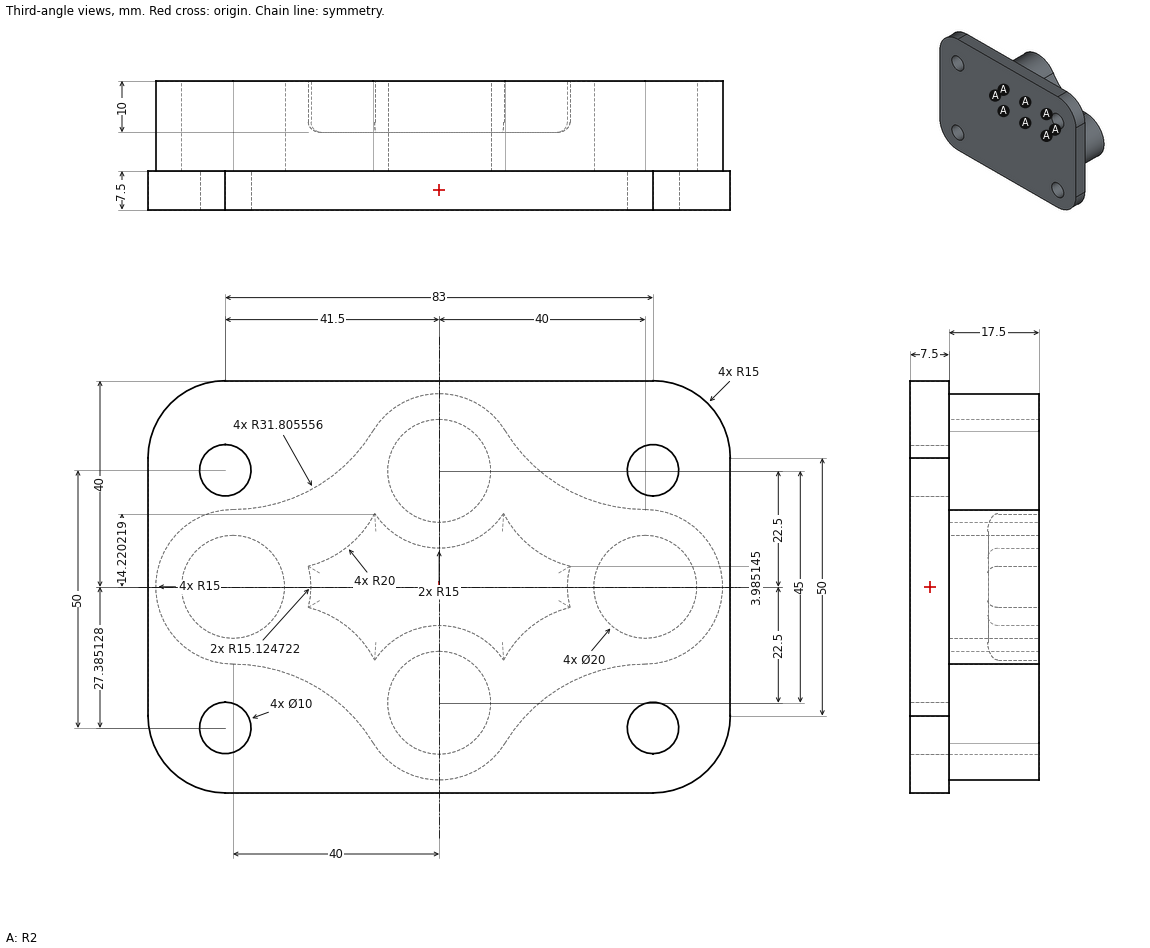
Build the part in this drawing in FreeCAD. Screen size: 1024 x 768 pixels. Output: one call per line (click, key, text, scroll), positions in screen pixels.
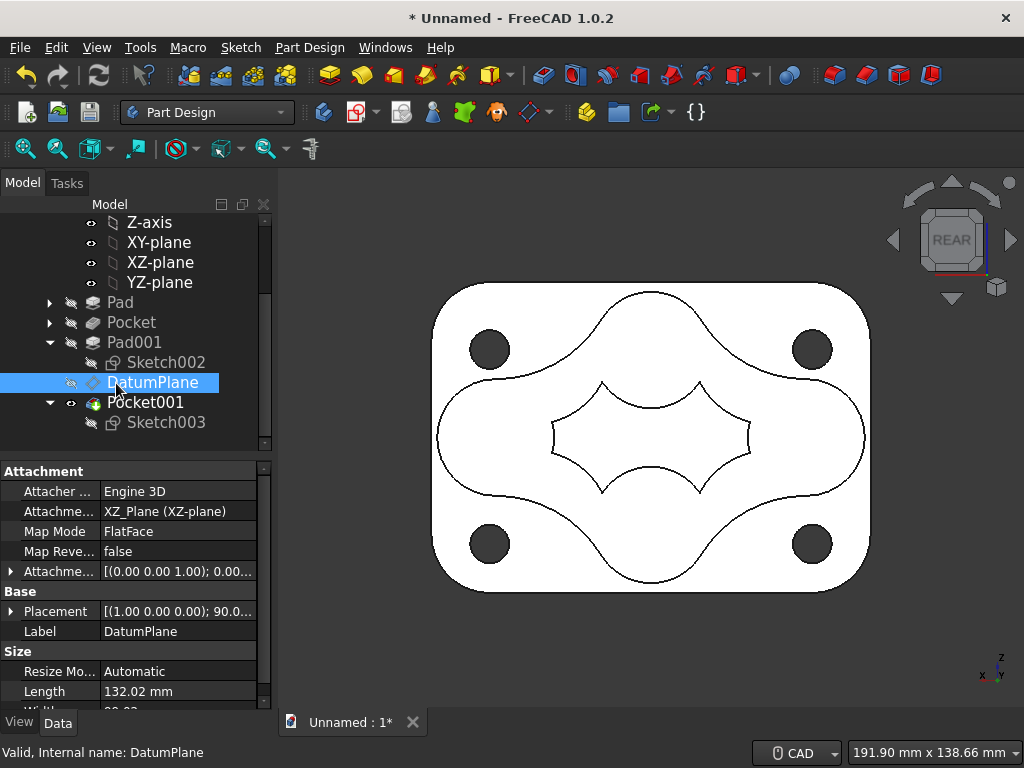
click(651, 353)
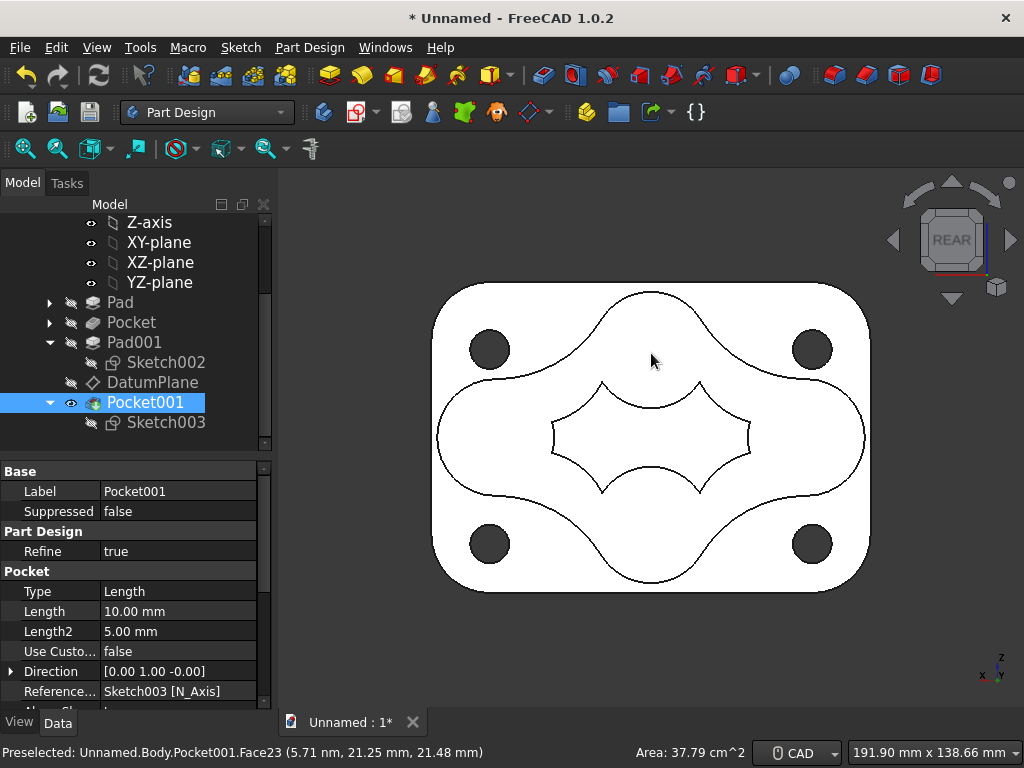
click(356, 112)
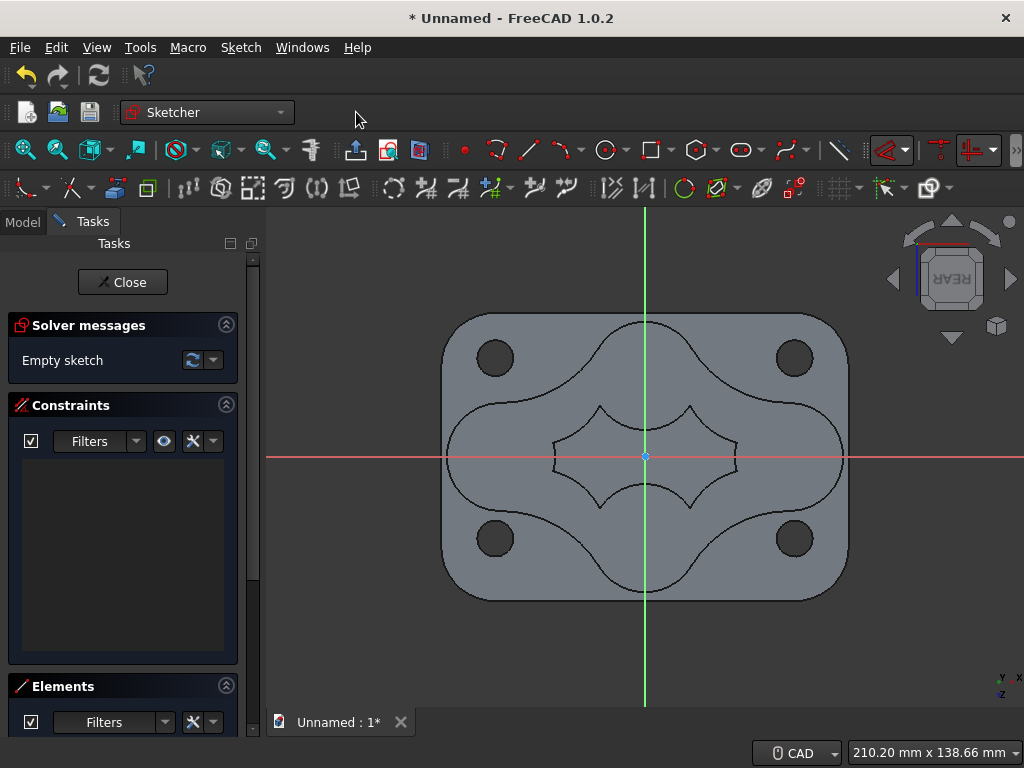
click(606, 150)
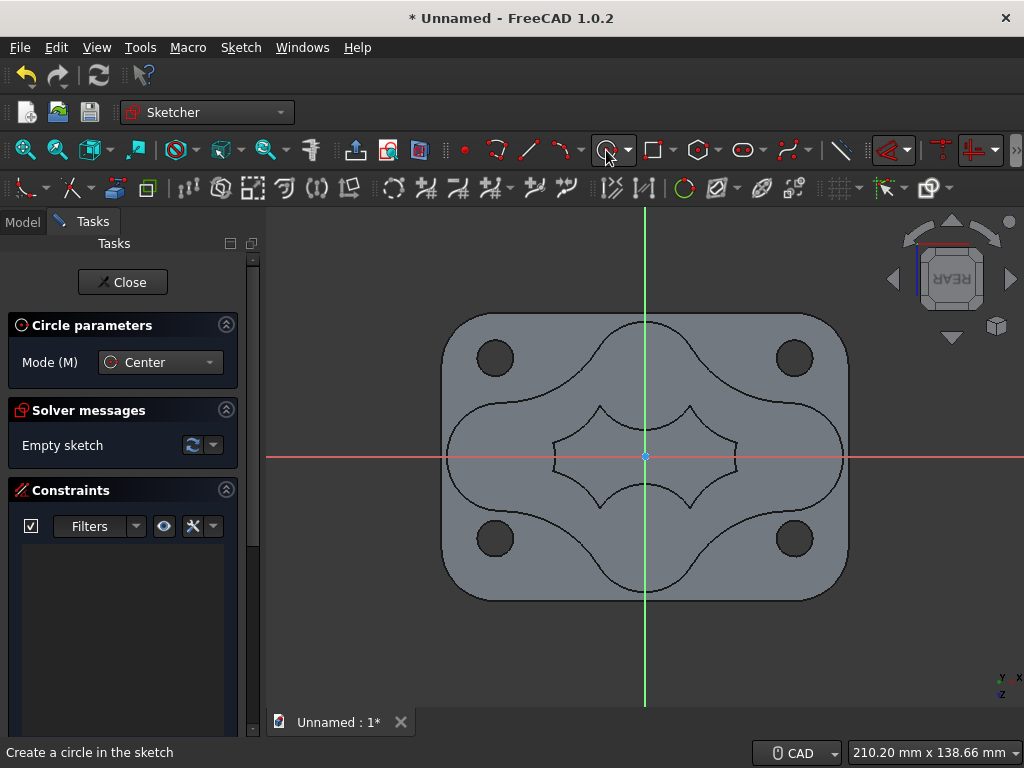
click(789, 457)
move(815, 432)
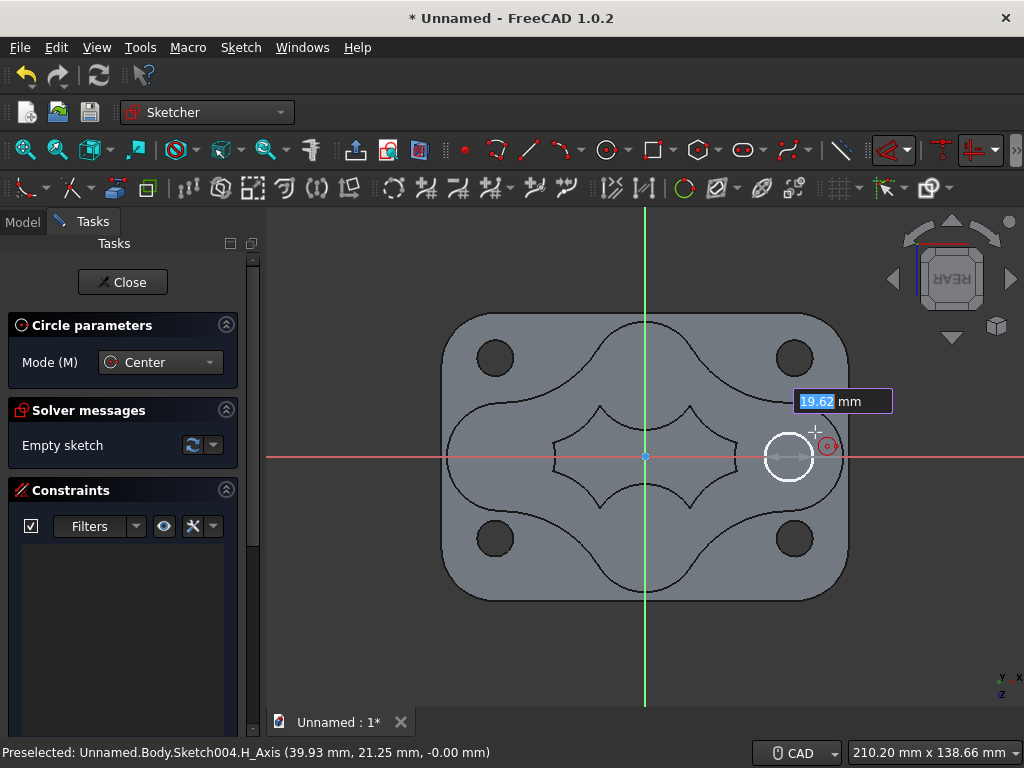
text(20)
key(Return)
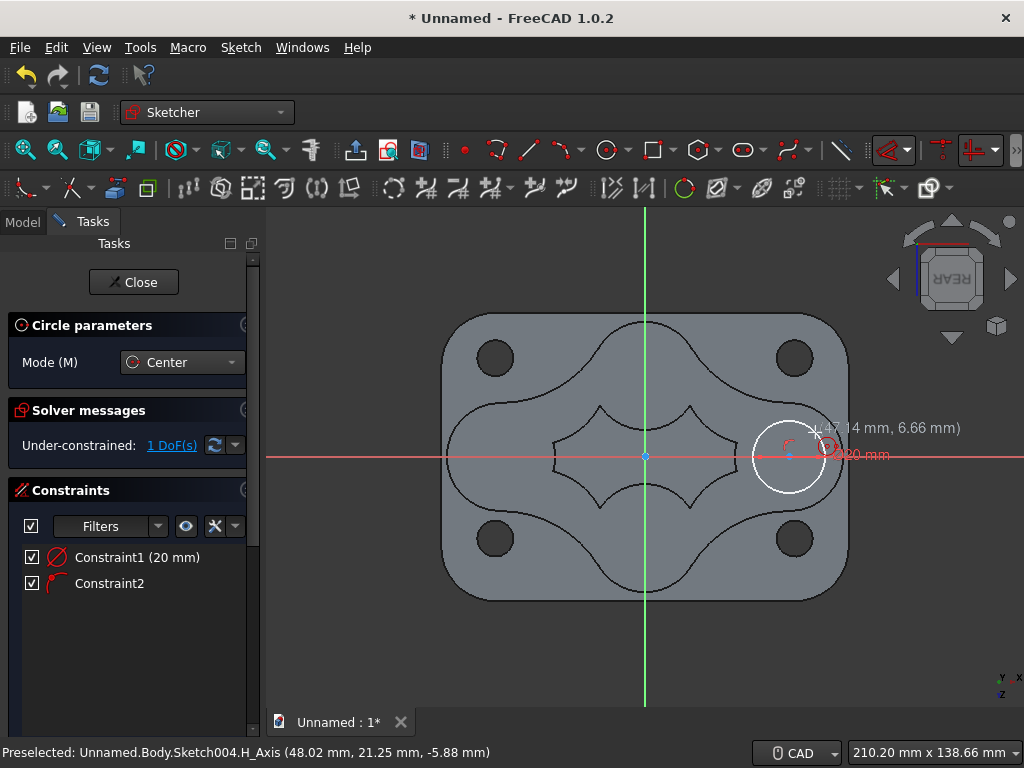
click(645, 538)
move(670, 513)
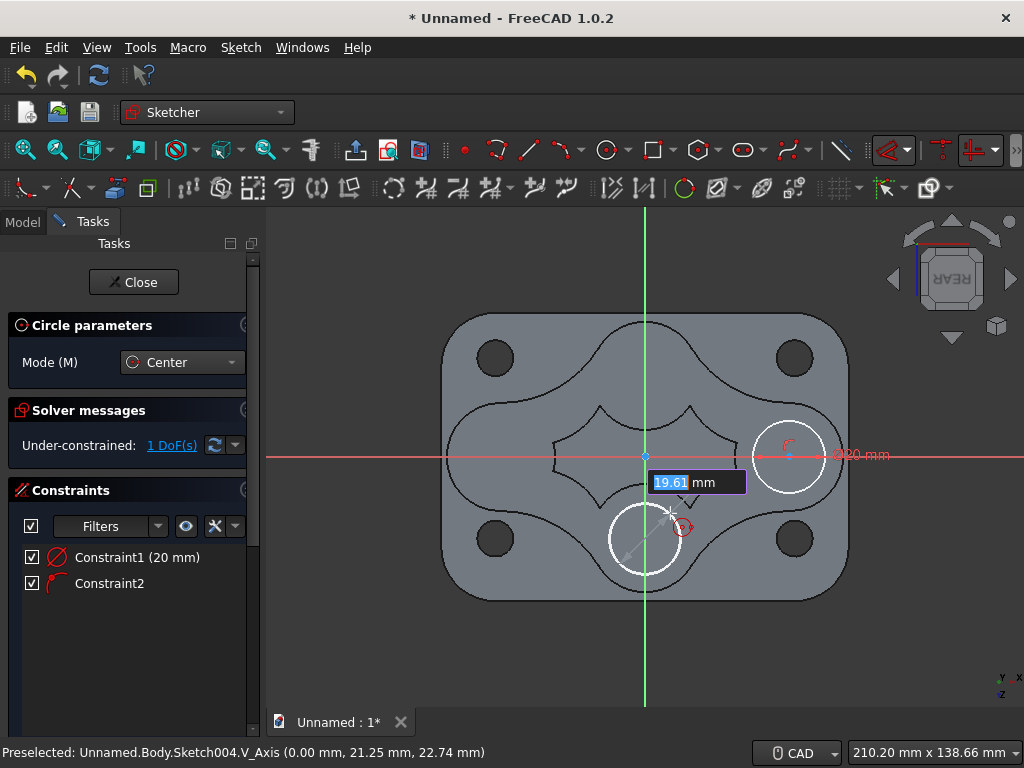
text(20)
key(Return)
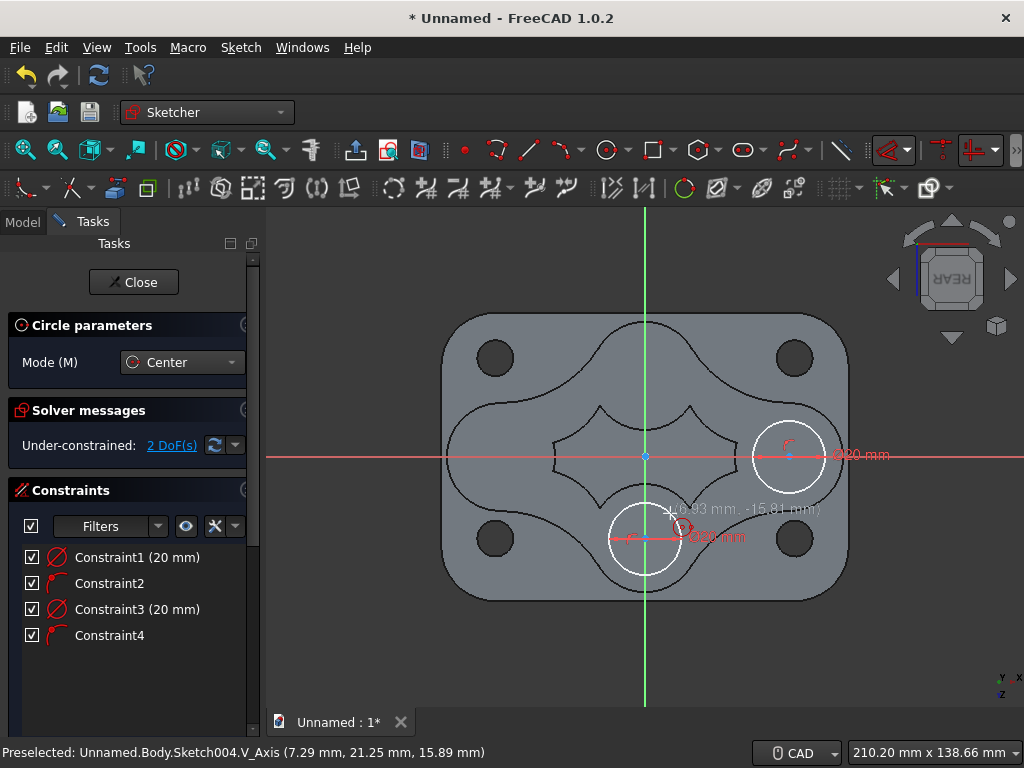
click(645, 376)
move(670, 350)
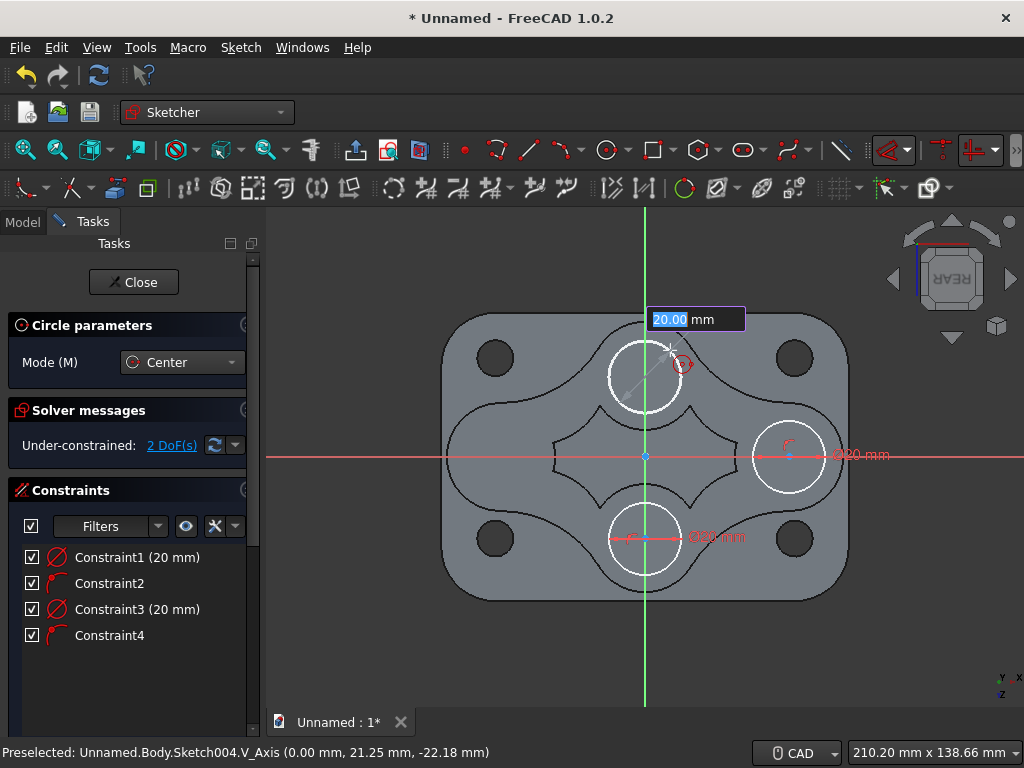
text(20)
key(Return)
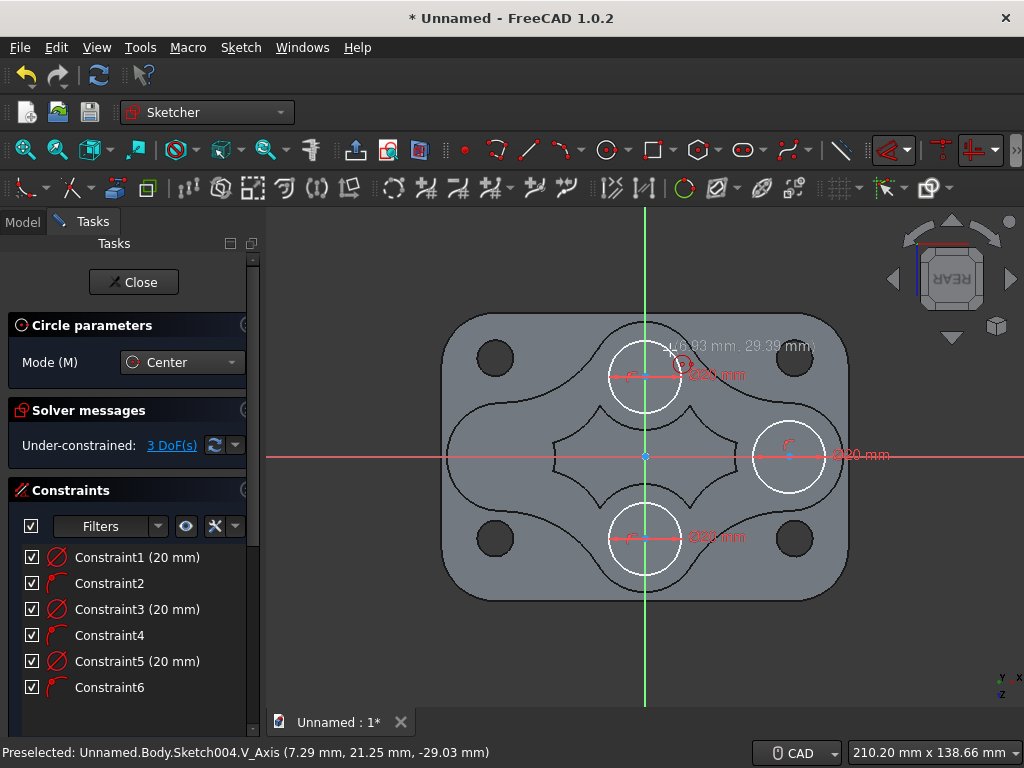
click(501, 457)
move(526, 432)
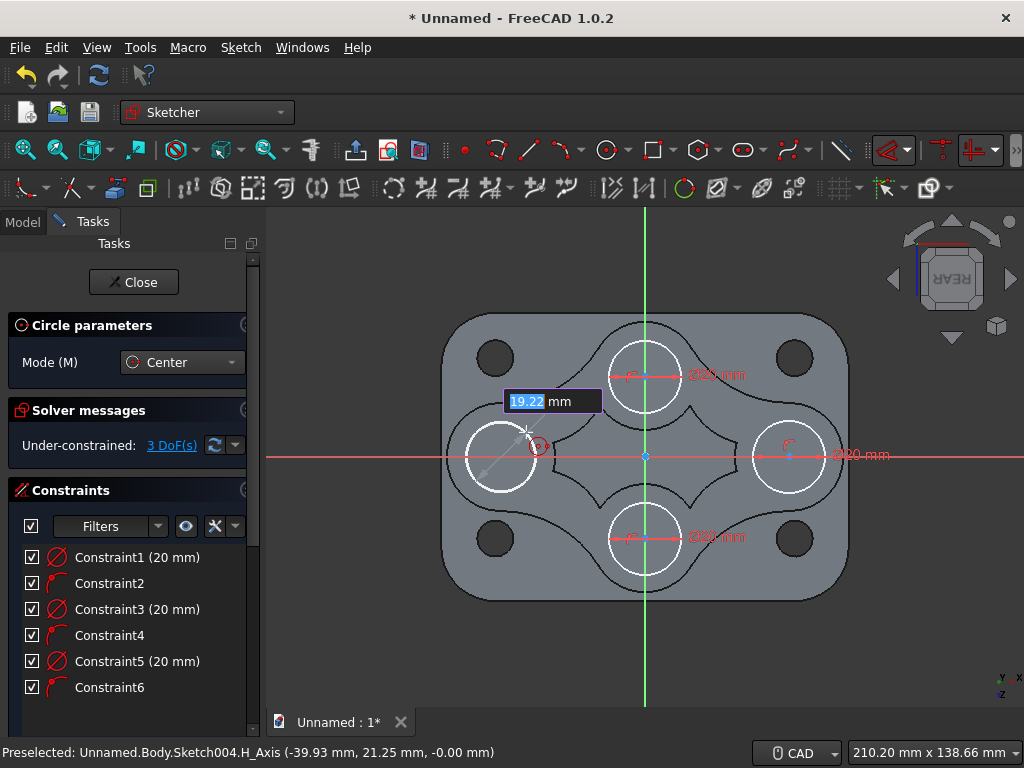
text(20)
key(Return)
key(Escape)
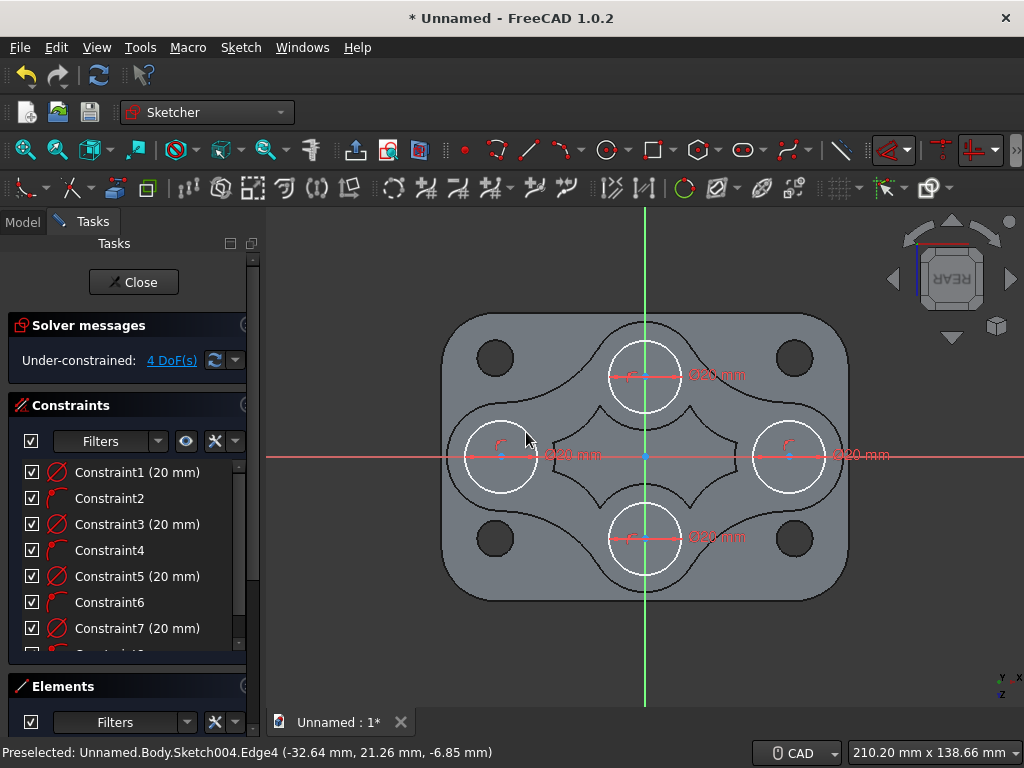
click(789, 457)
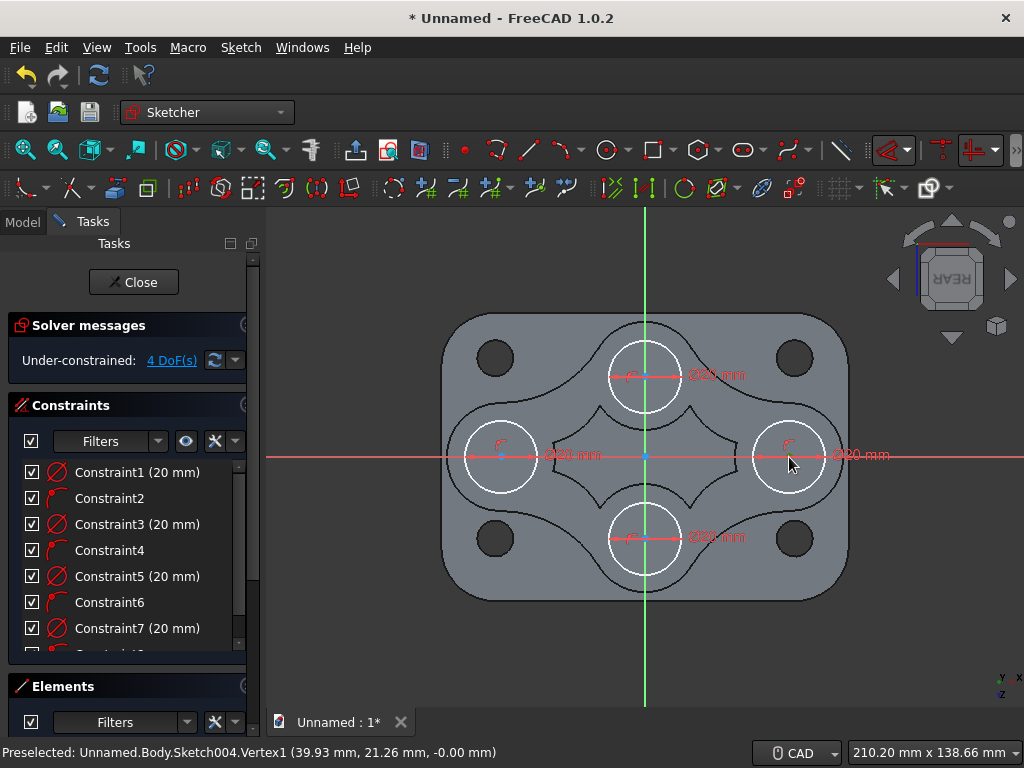
click(910, 150)